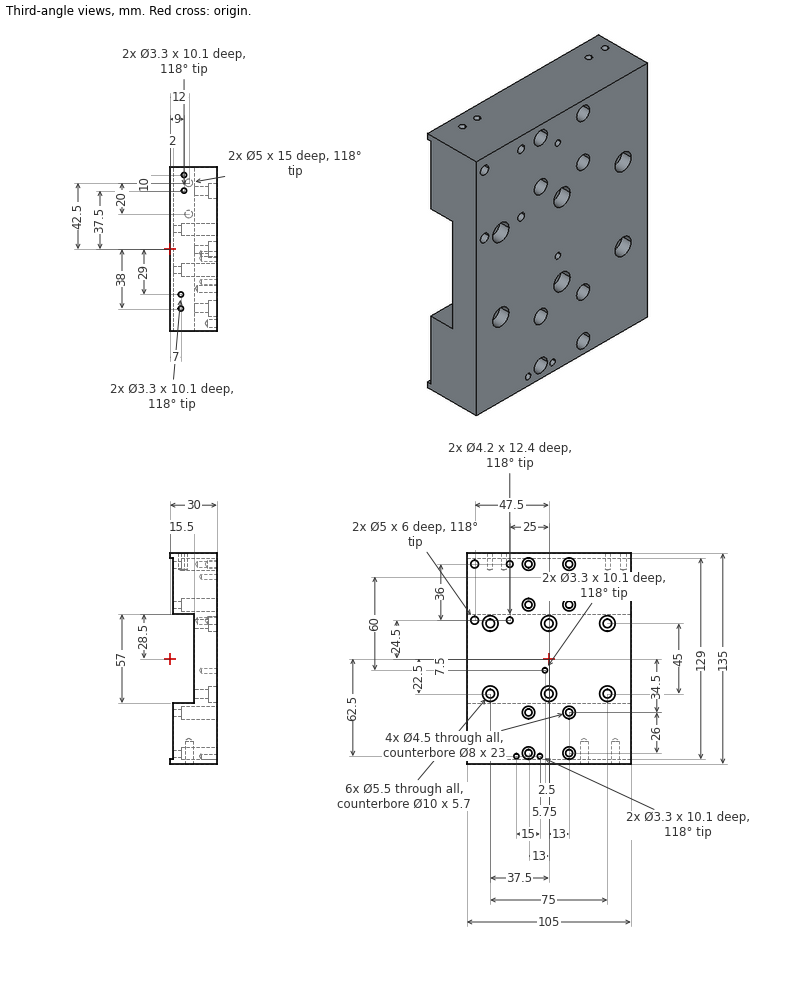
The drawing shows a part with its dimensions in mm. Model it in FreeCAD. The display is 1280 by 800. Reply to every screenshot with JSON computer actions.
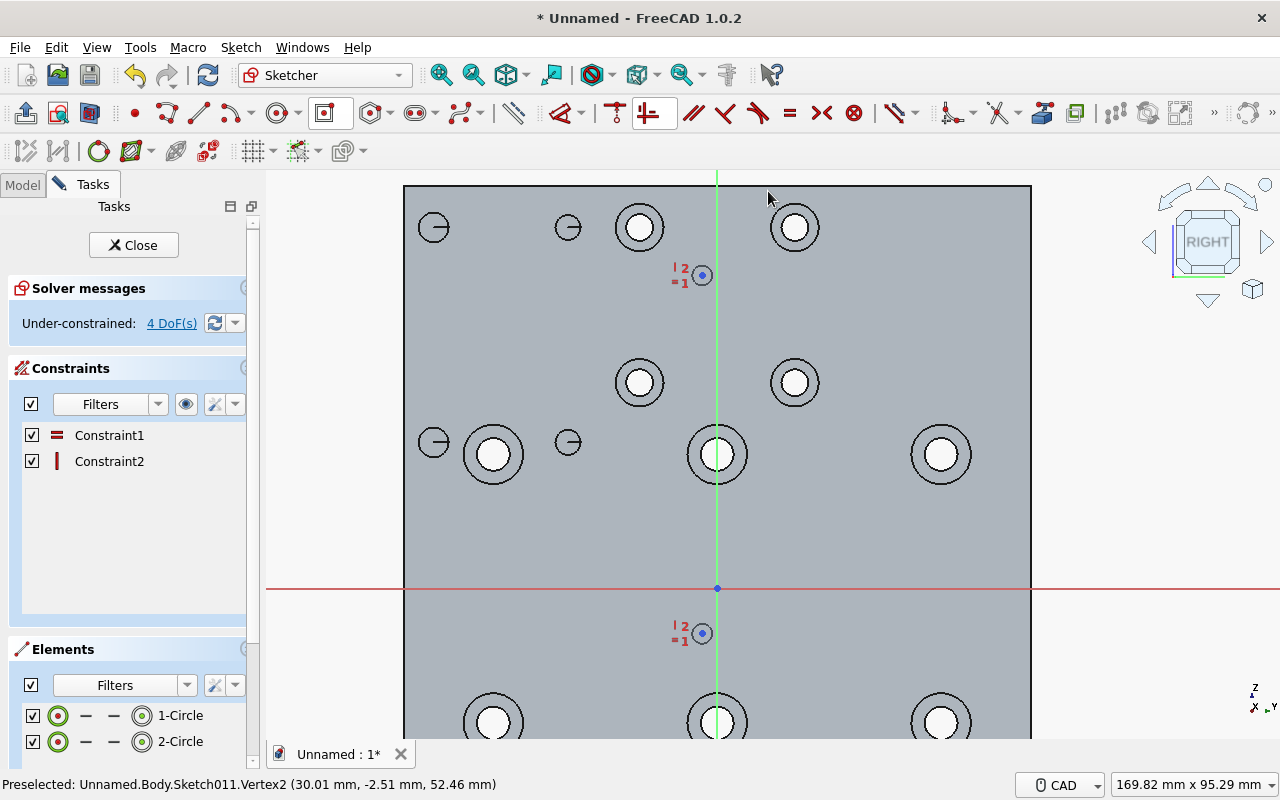
{"action": "left_click", "coordinate": [560, 114]}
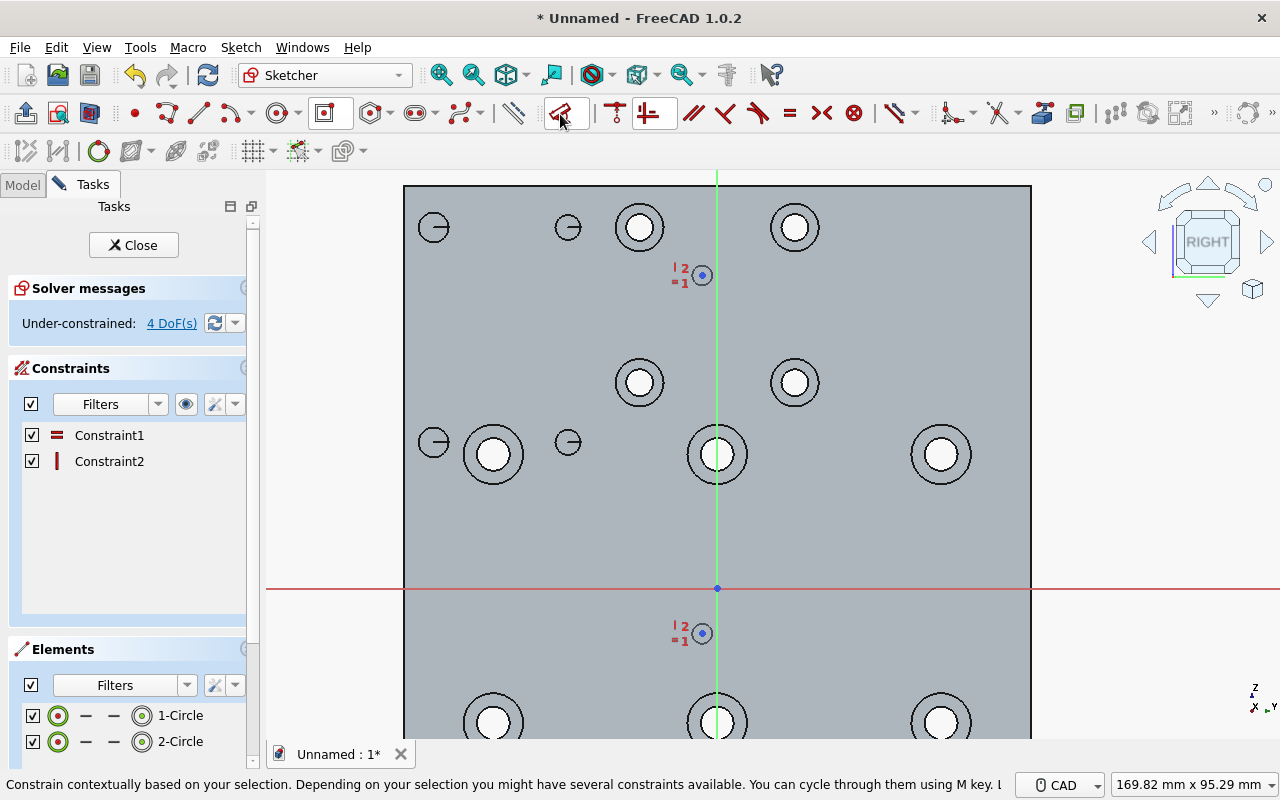
{"action": "scroll", "coordinate": [695, 627], "scroll_direction": "up", "scroll_amount": 4}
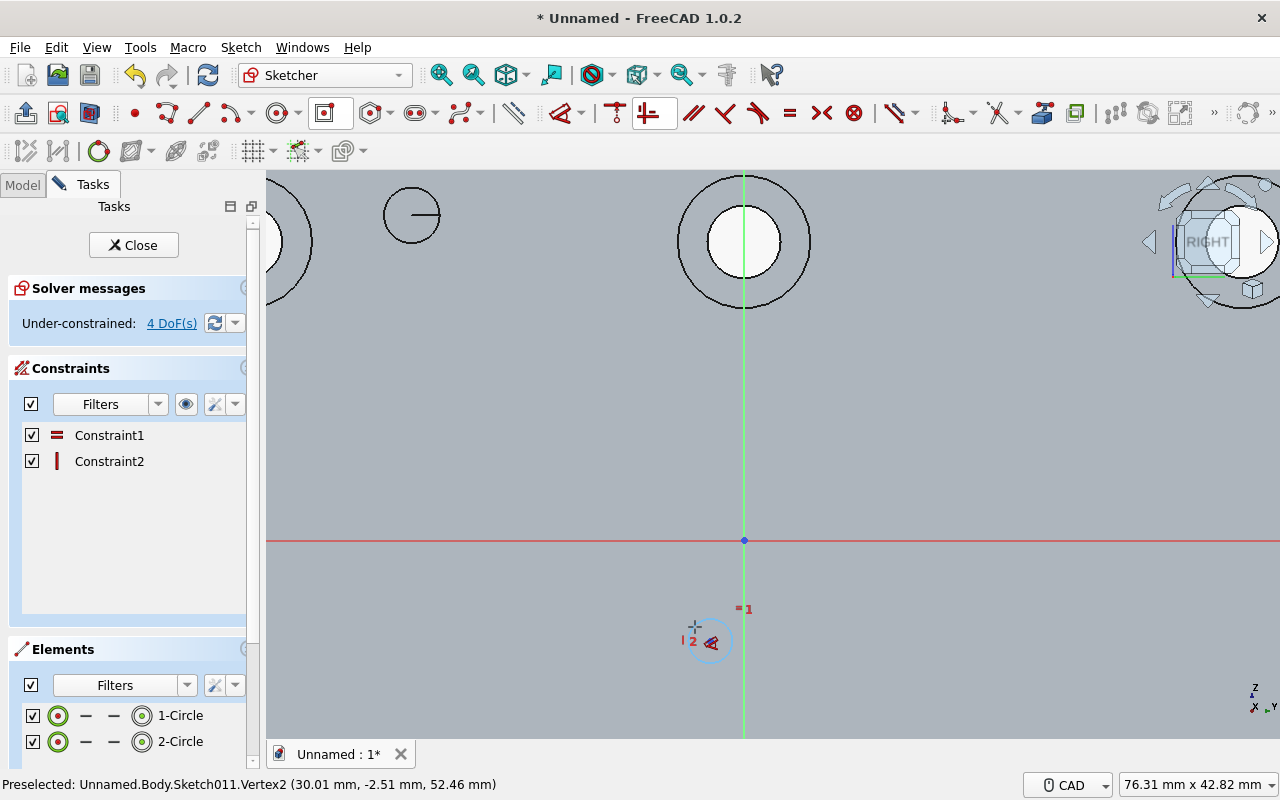
{"action": "left_click", "coordinate": [695, 626]}
{"action": "left_click", "coordinate": [672, 604]}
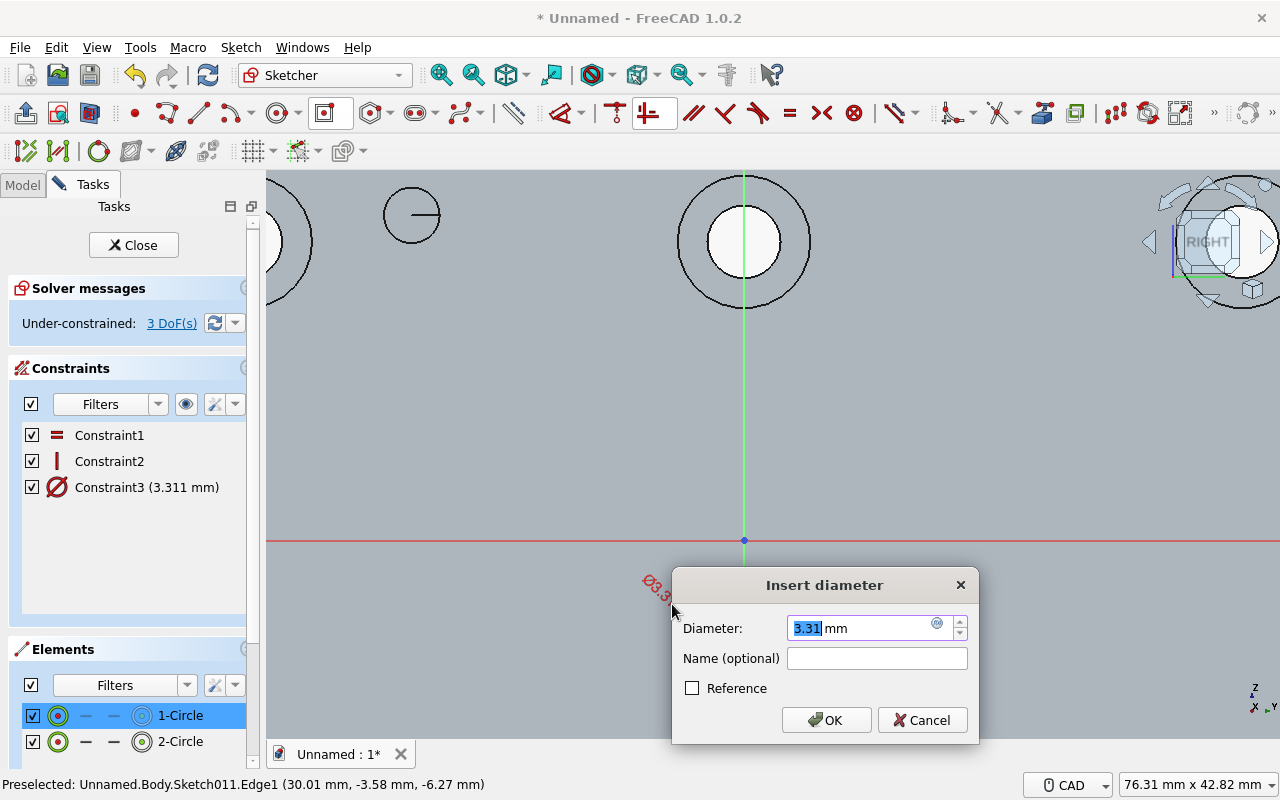
{"action": "type", "text": "3.3"}
{"action": "key", "text": "Return"}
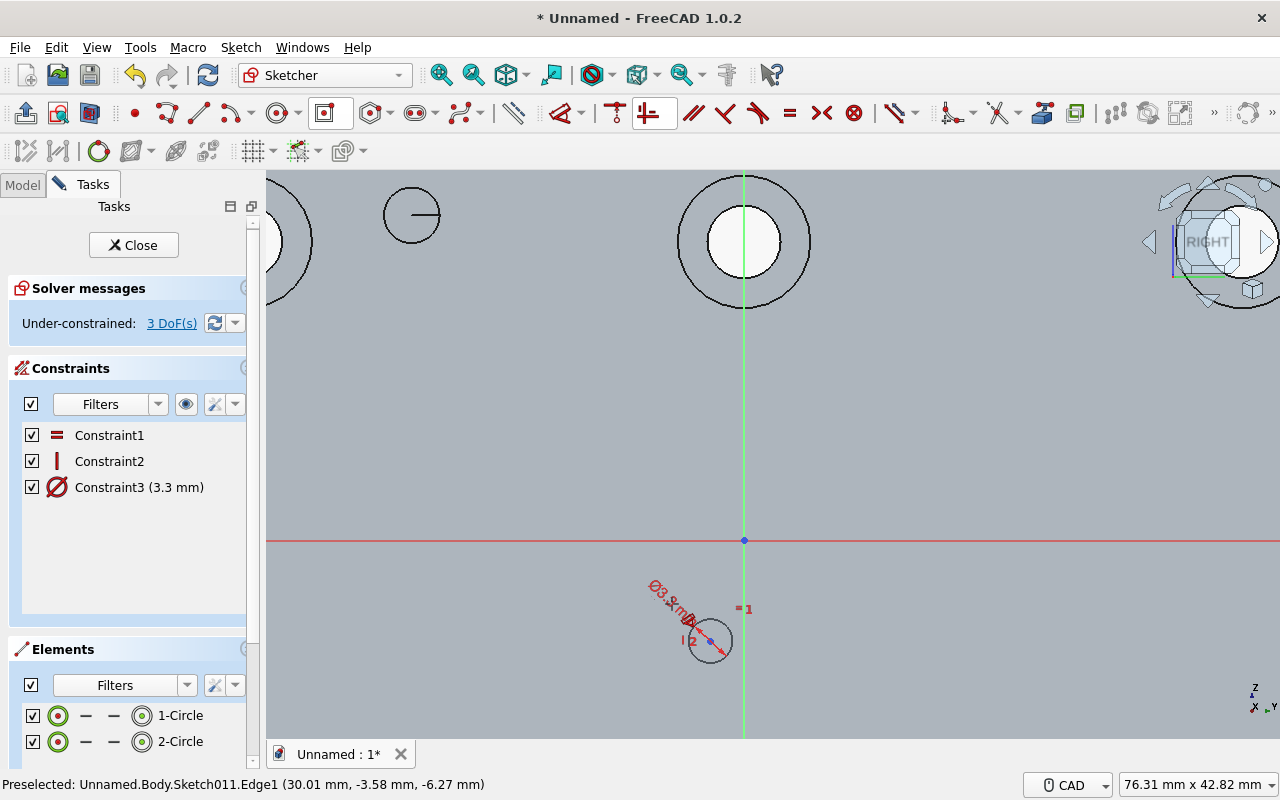
{"action": "left_click", "coordinate": [710, 641]}
{"action": "left_click", "coordinate": [727, 675]}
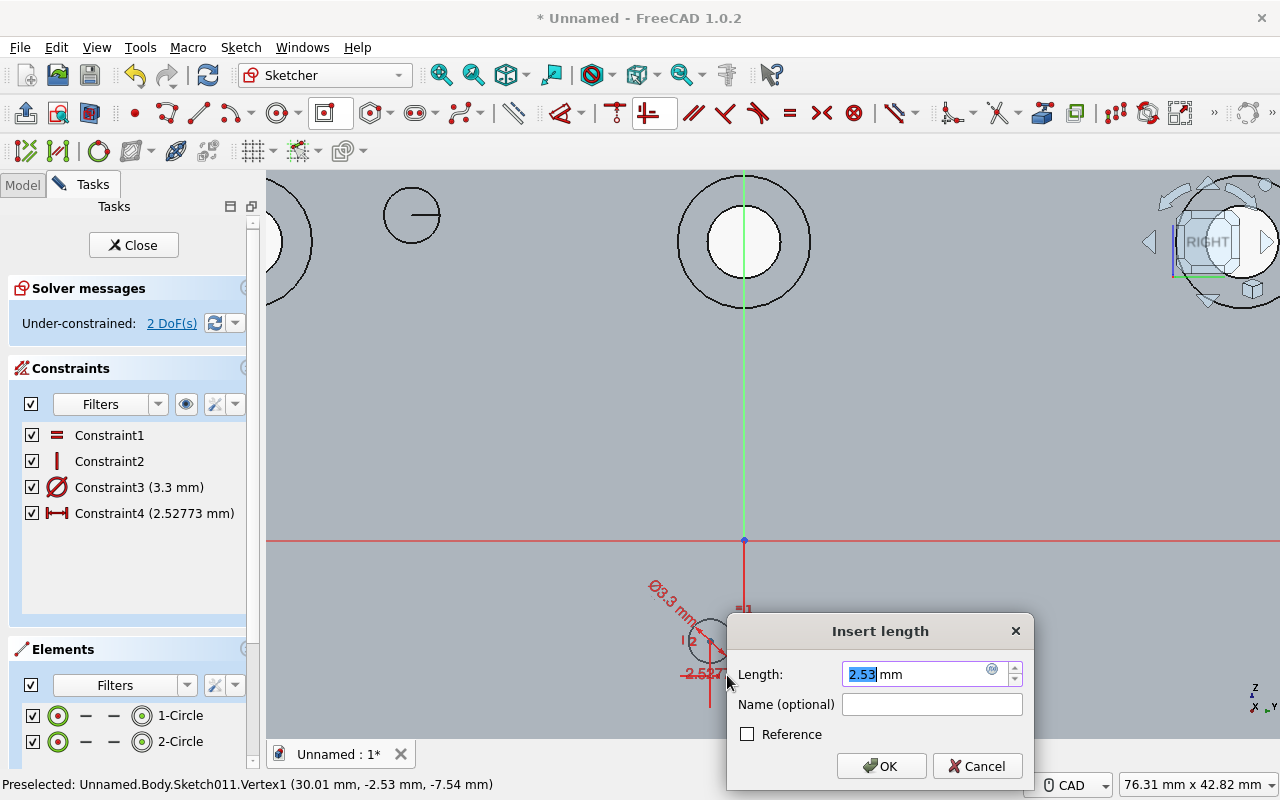
{"action": "type", "text": "2.5"}
{"action": "key", "text": "Return"}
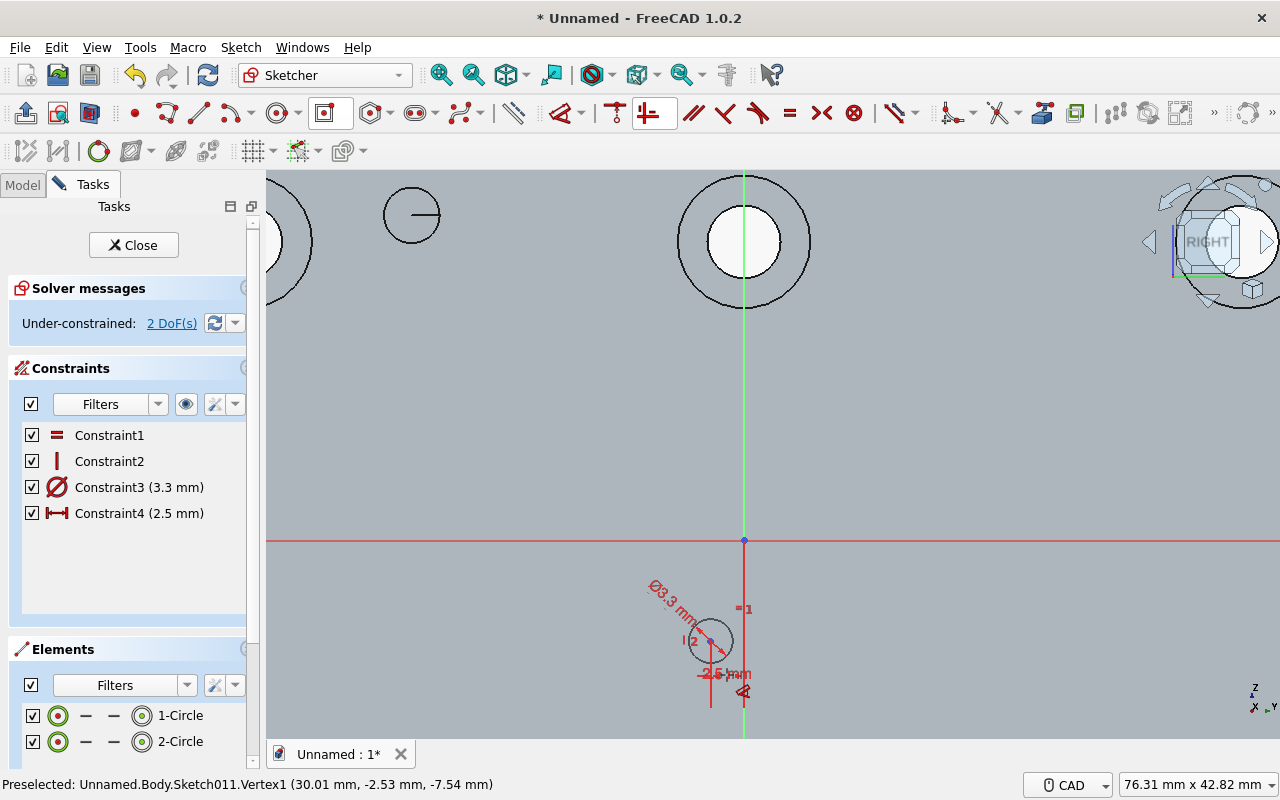
{"action": "left_click", "coordinate": [711, 641]}
{"action": "left_click", "coordinate": [778, 591]}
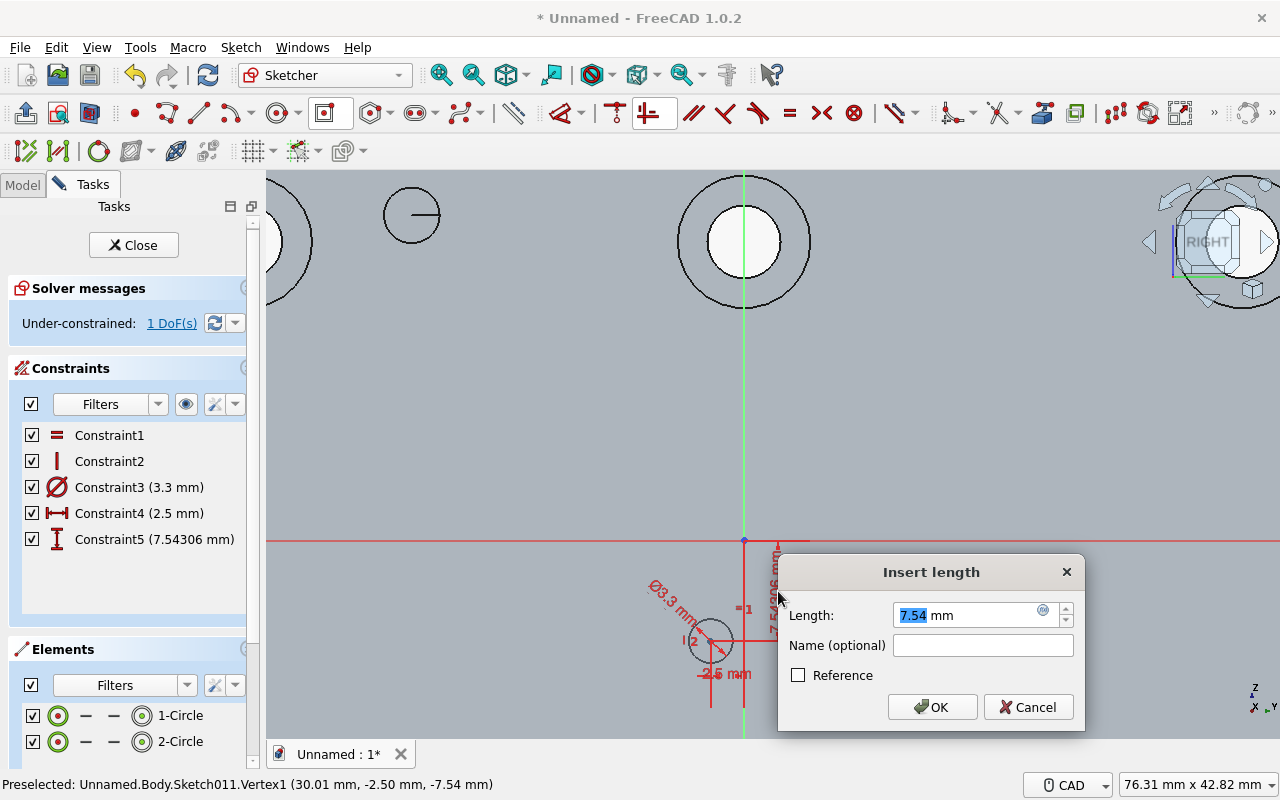
{"action": "type", "text": "7.5"}
{"action": "key", "text": "Return"}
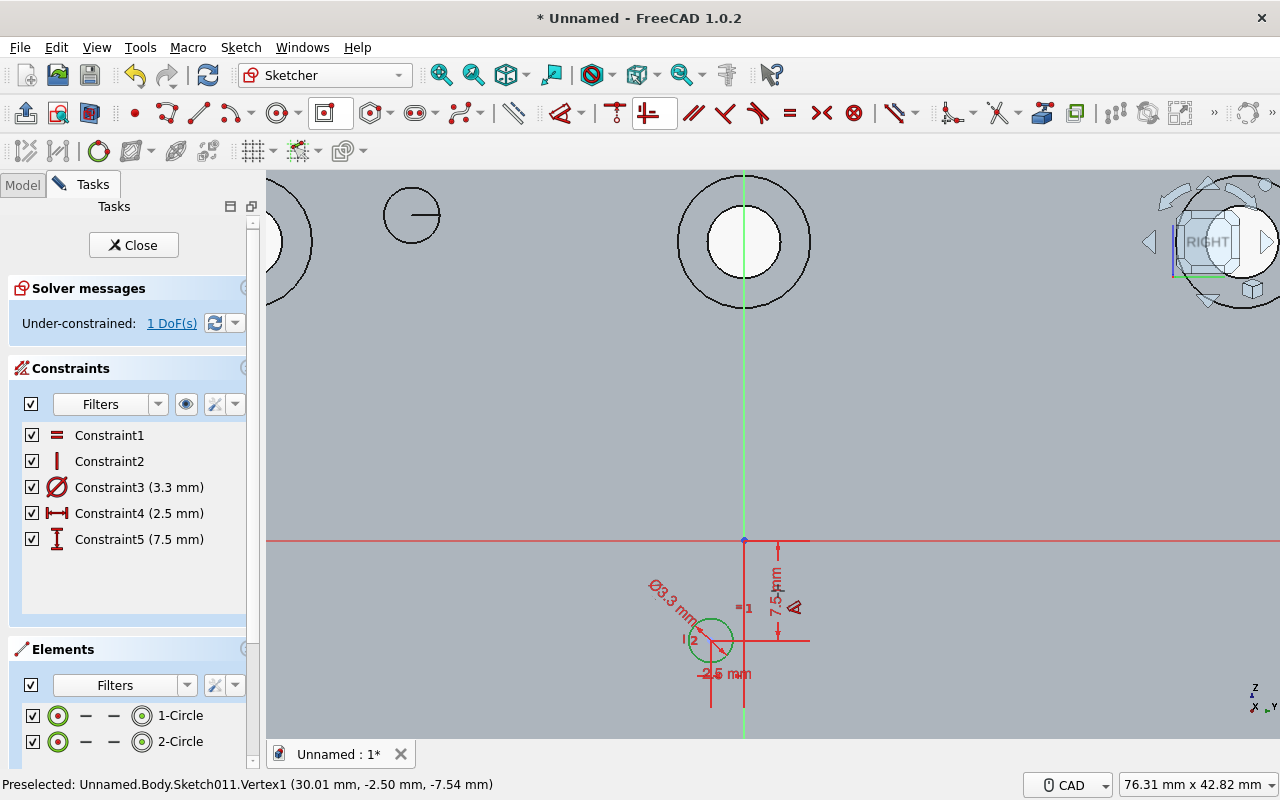
{"action": "left_click", "coordinate": [711, 641]}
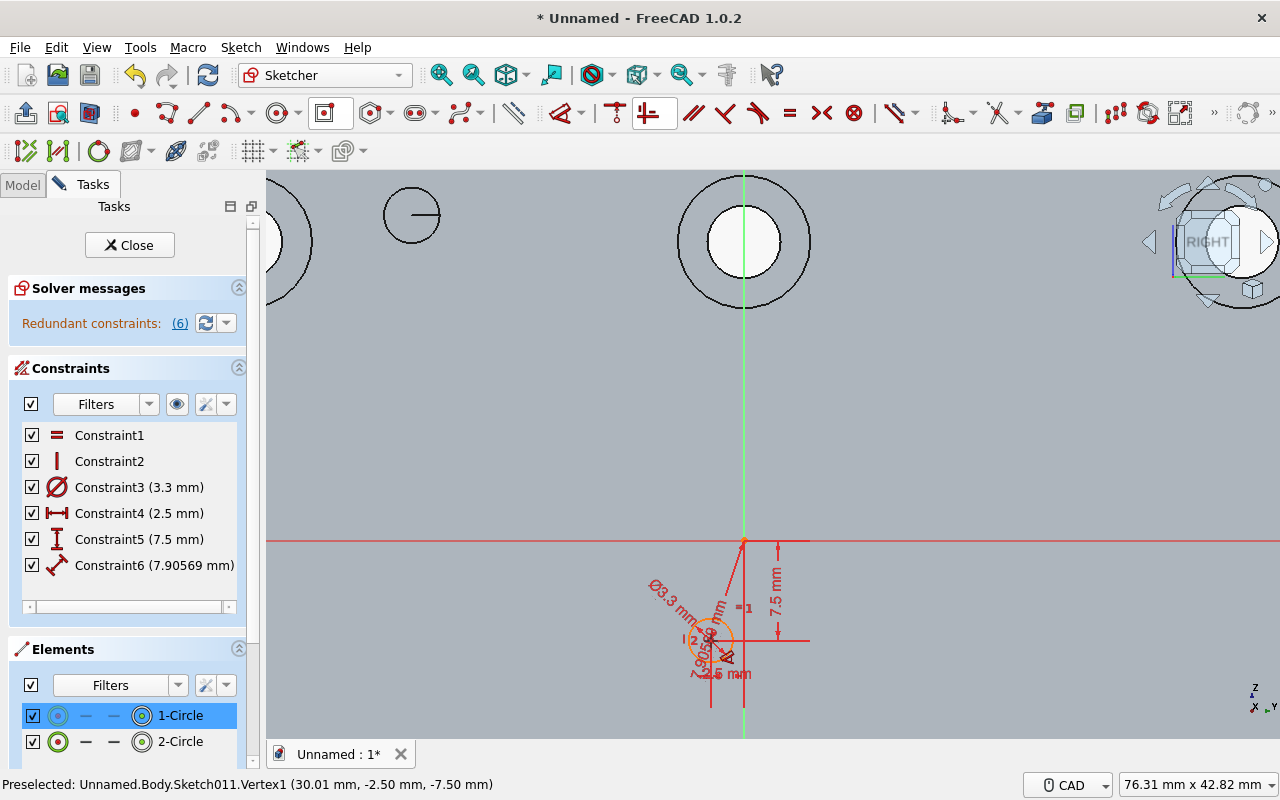
{"action": "scroll", "coordinate": [695, 628], "scroll_direction": "down", "scroll_amount": 4}